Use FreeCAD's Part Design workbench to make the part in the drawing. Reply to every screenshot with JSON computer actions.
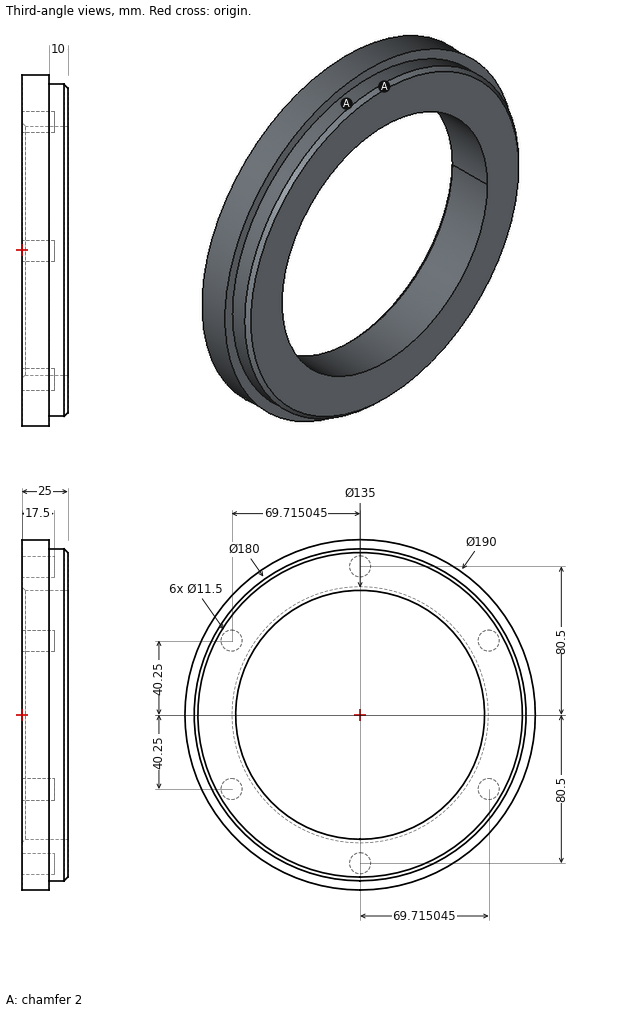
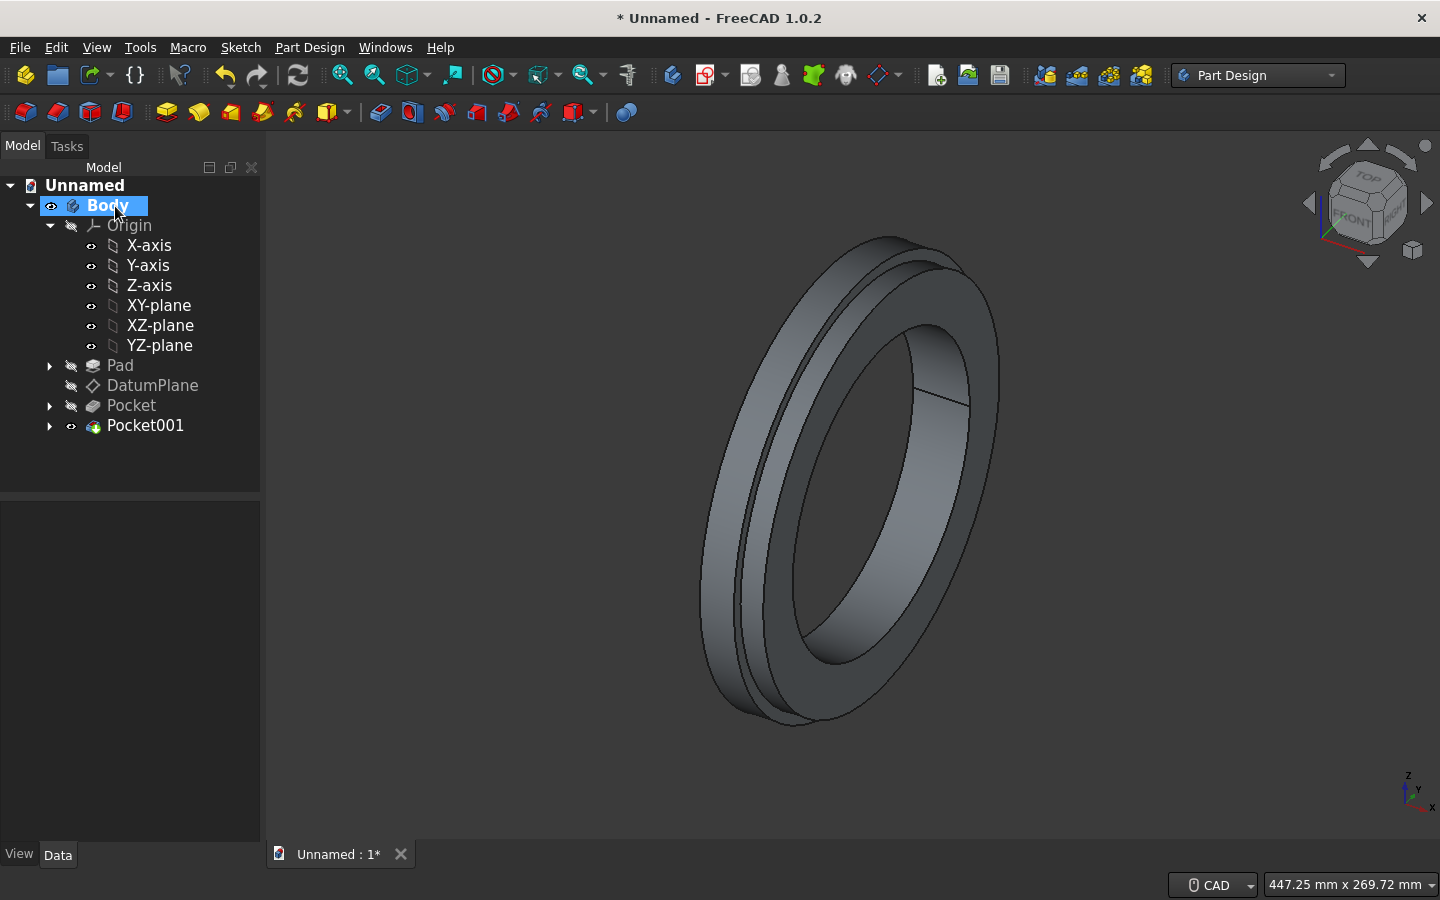
{"action": "left_click", "coordinate": [763, 611]}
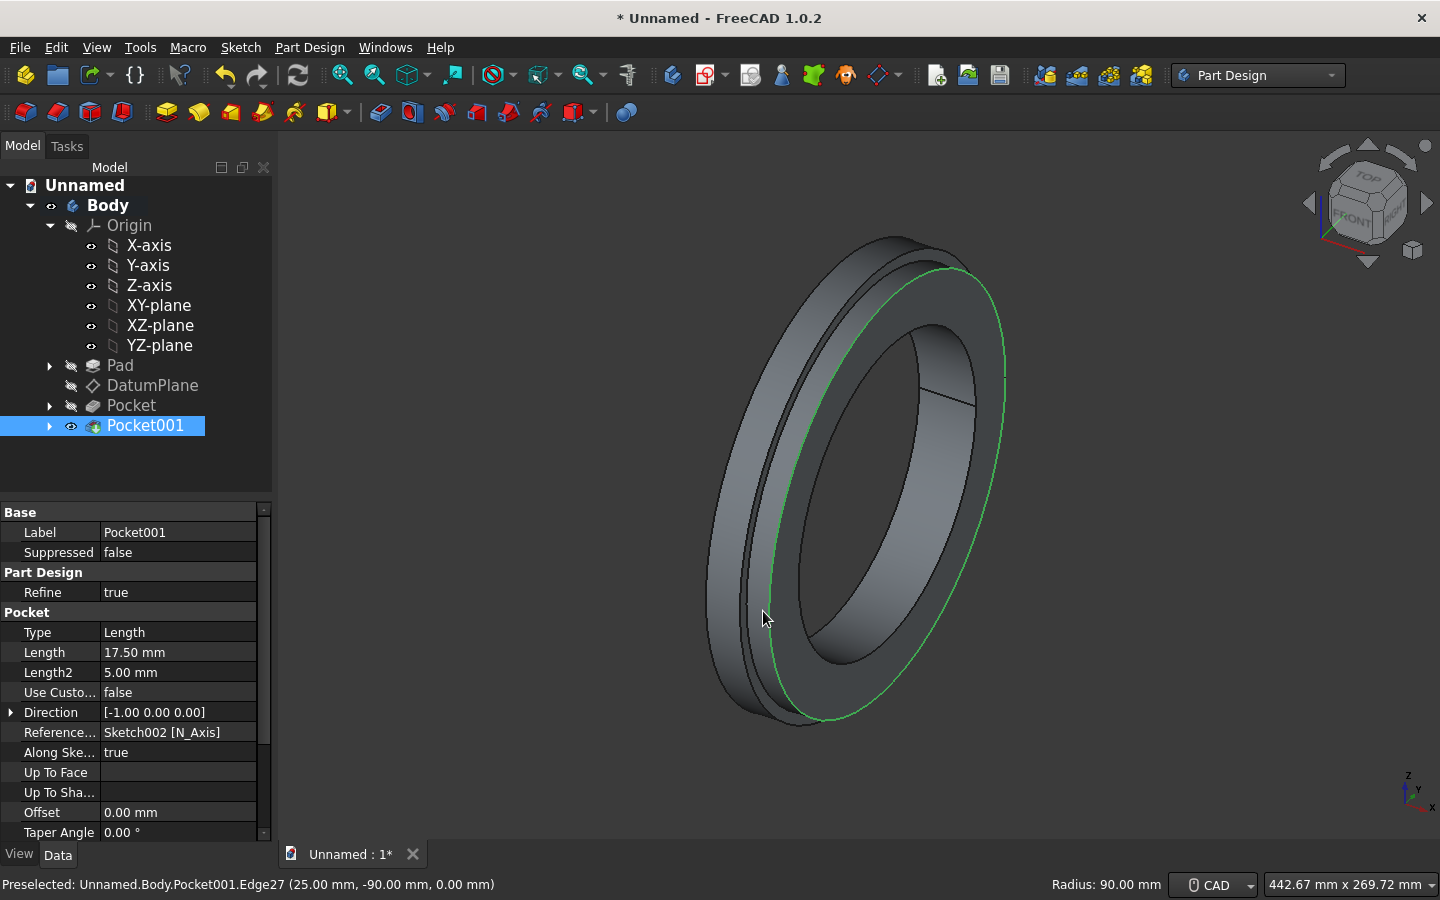
{"action": "key", "text": "0"}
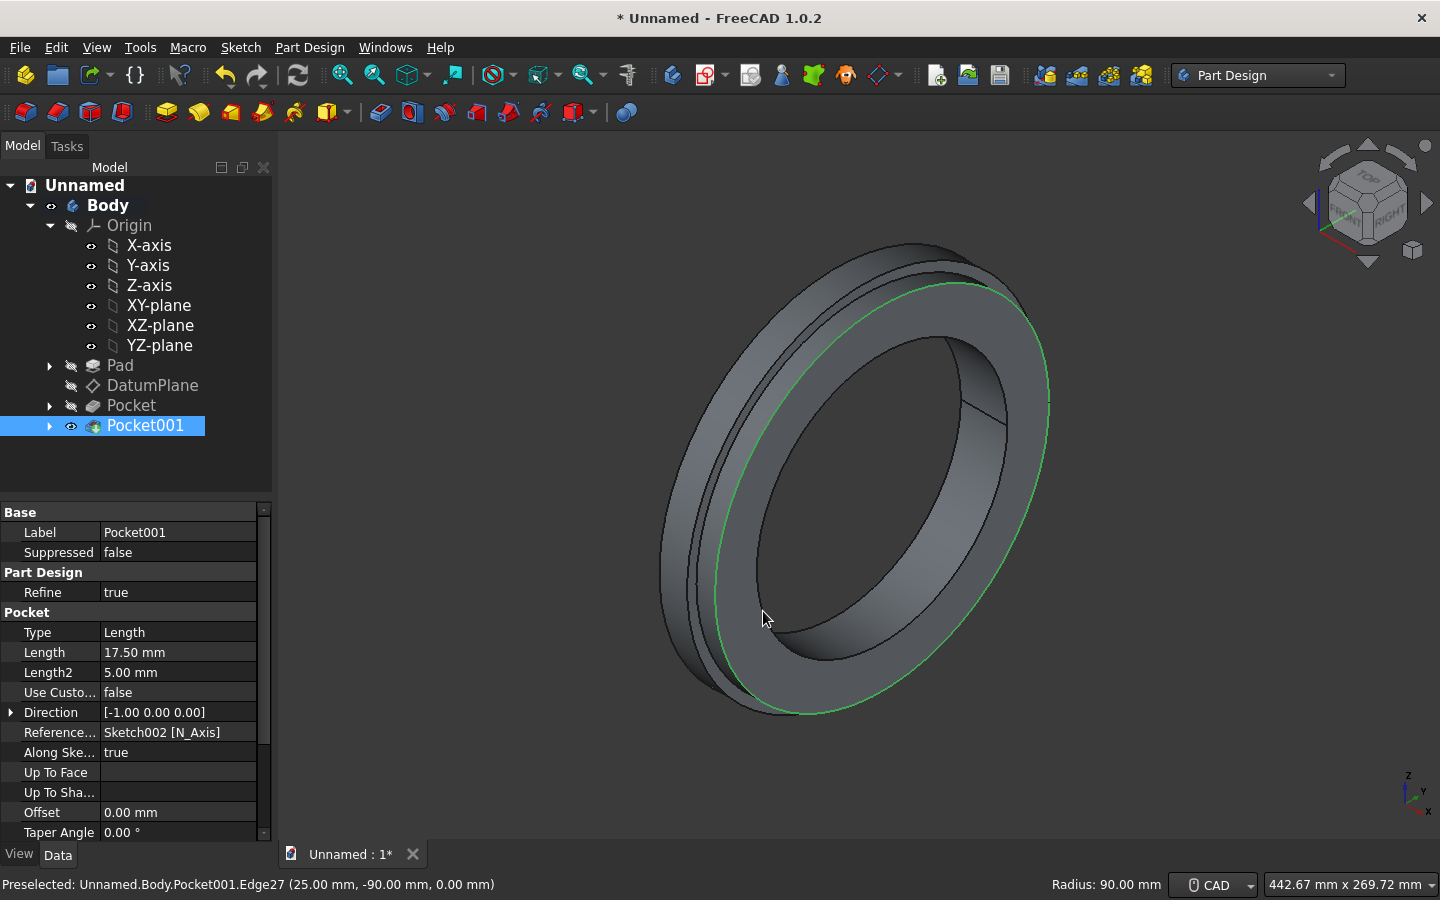
{"action": "key", "text": "2"}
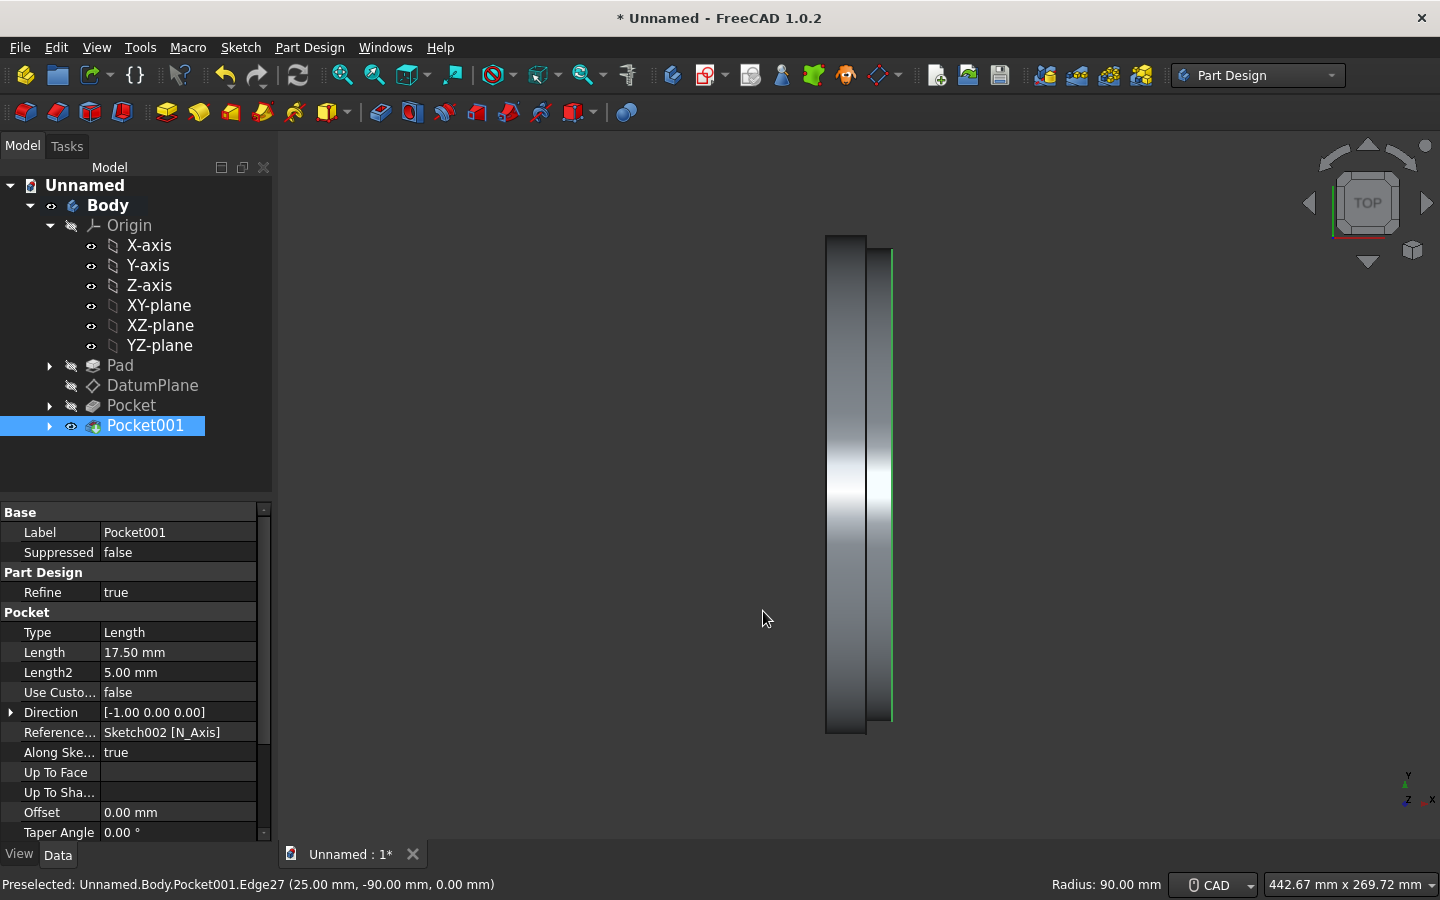
{"action": "key", "text": "1"}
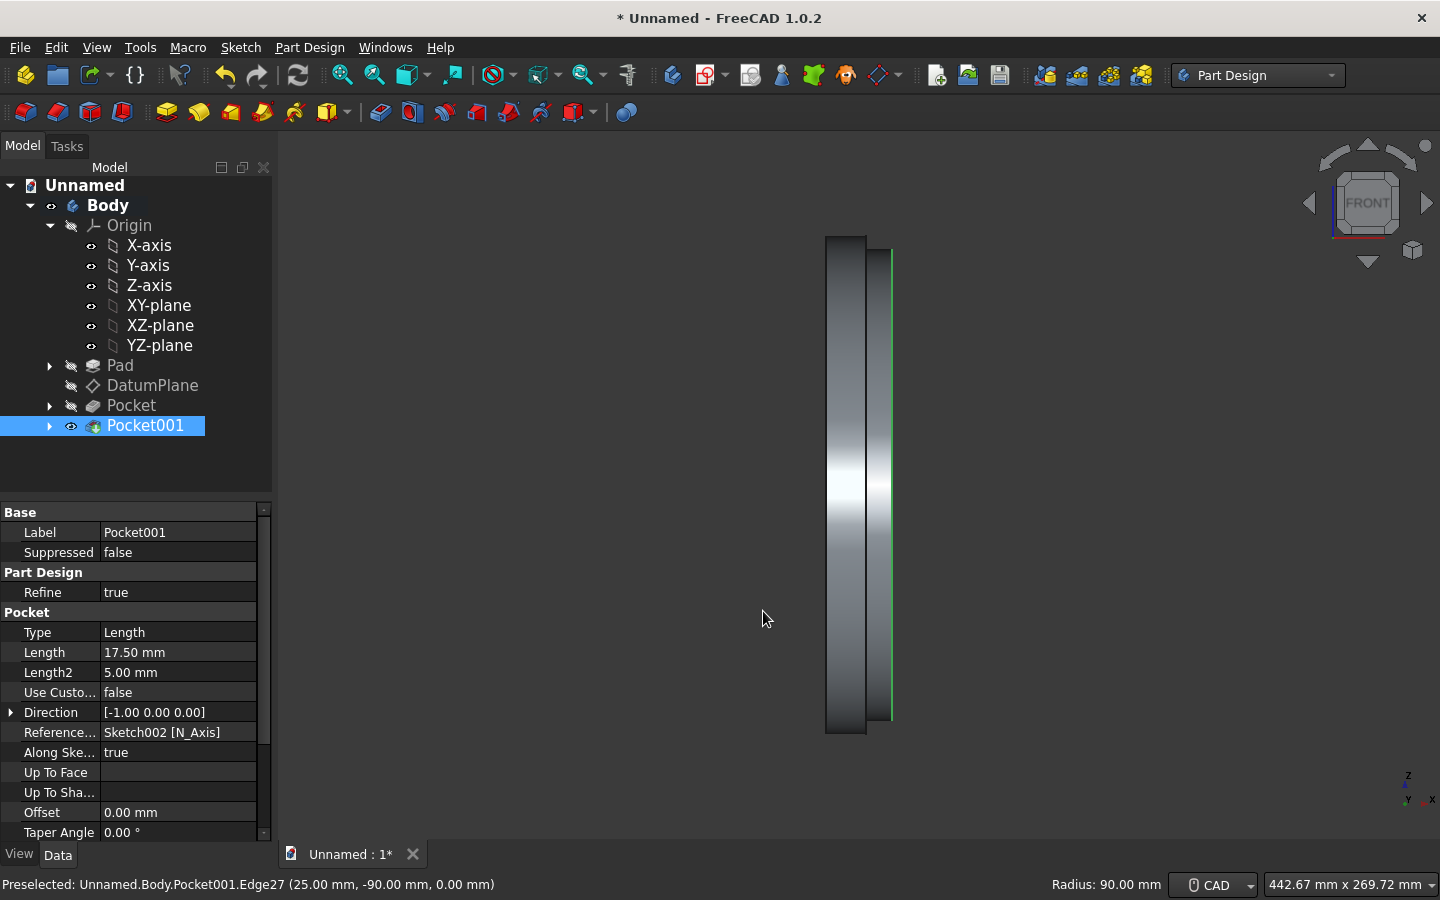
{"action": "key", "text": "3"}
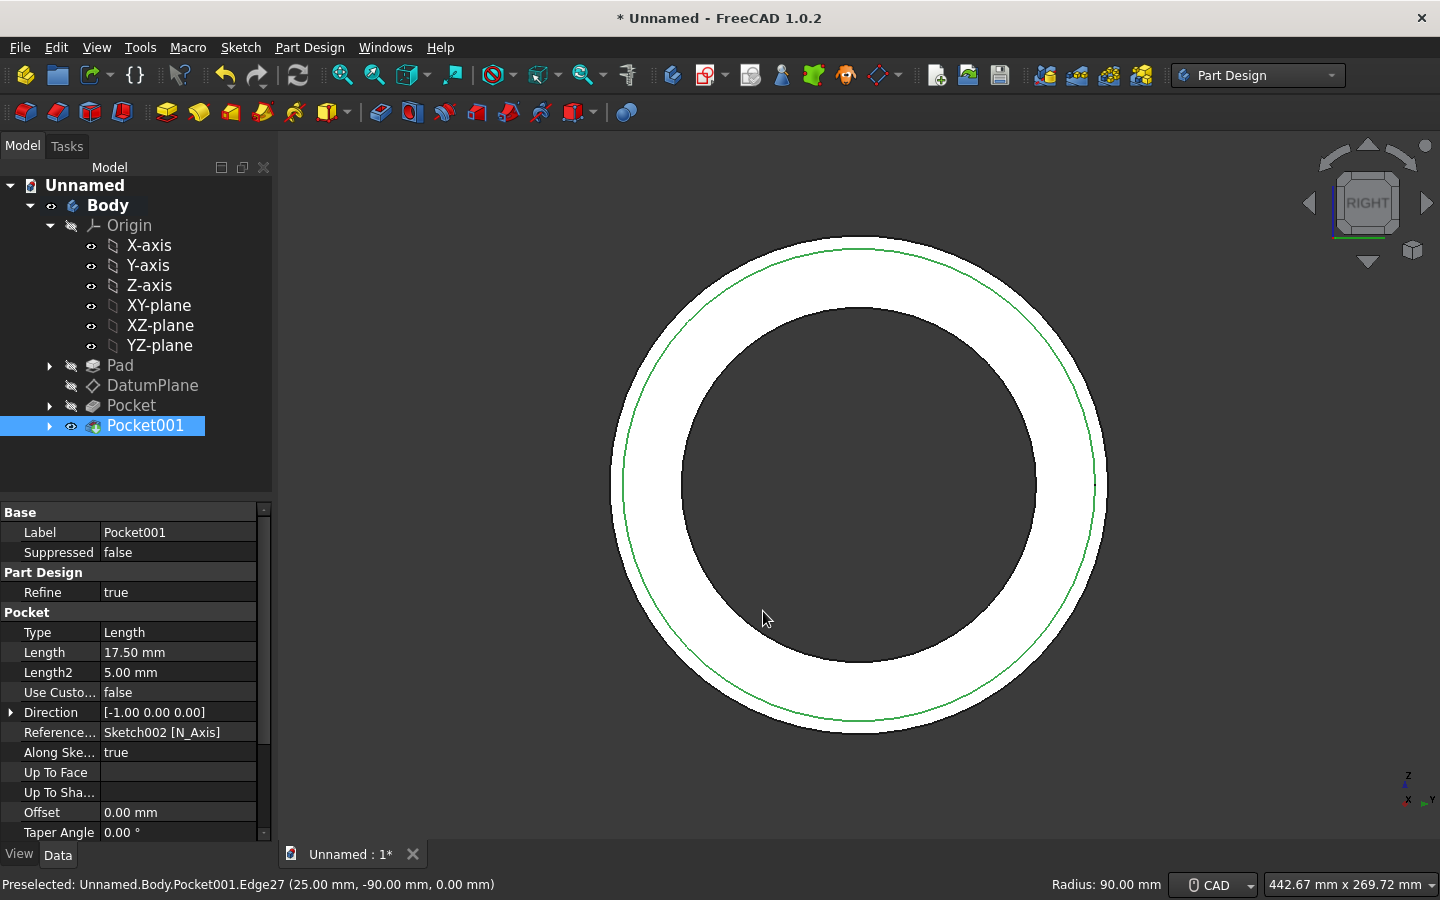
{"action": "key", "text": "5"}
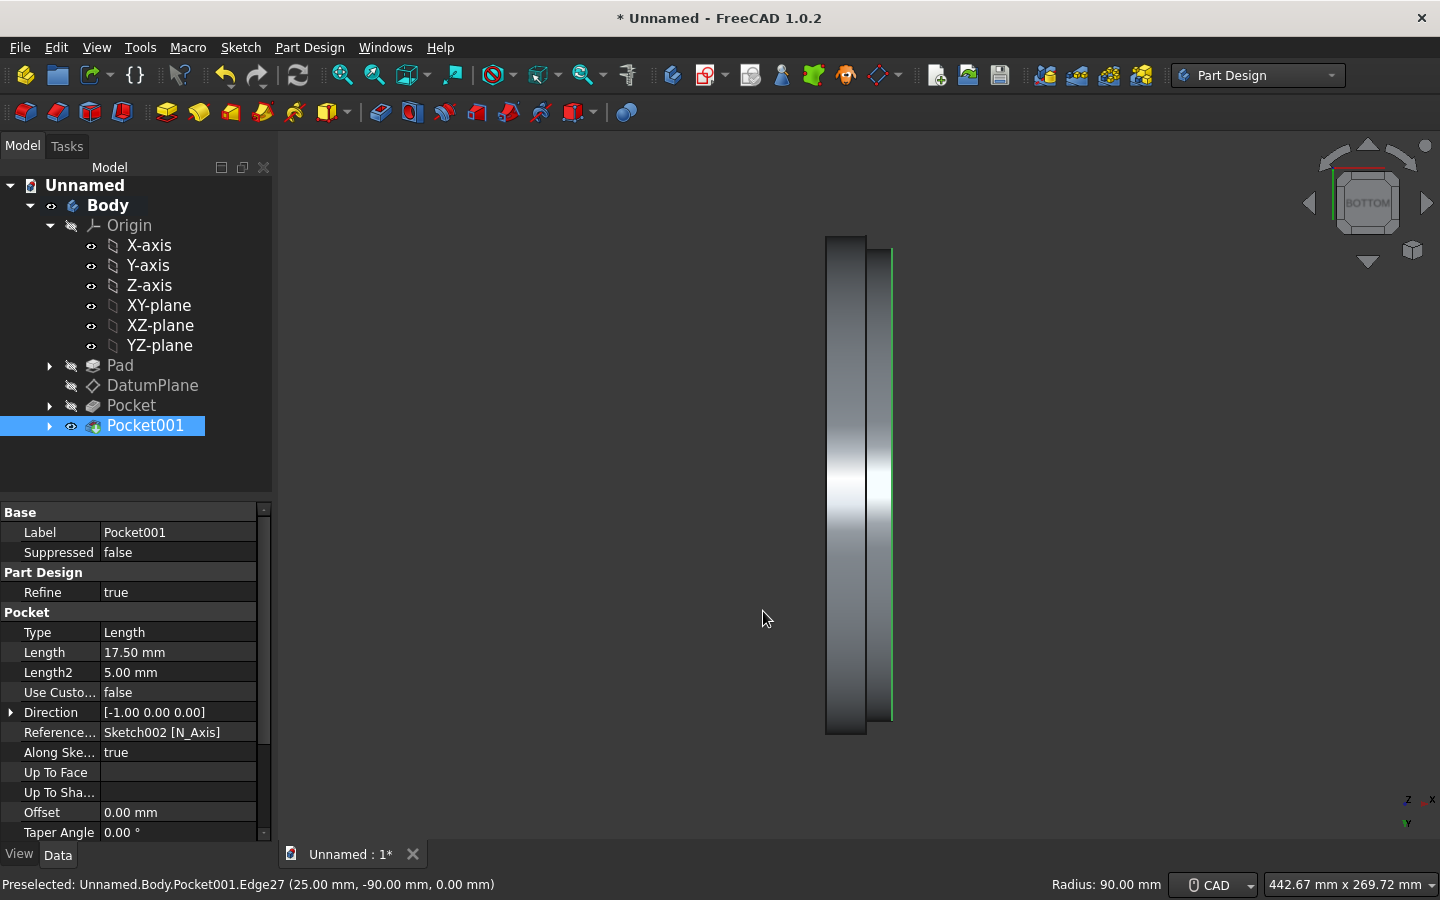
{"action": "key", "text": "4"}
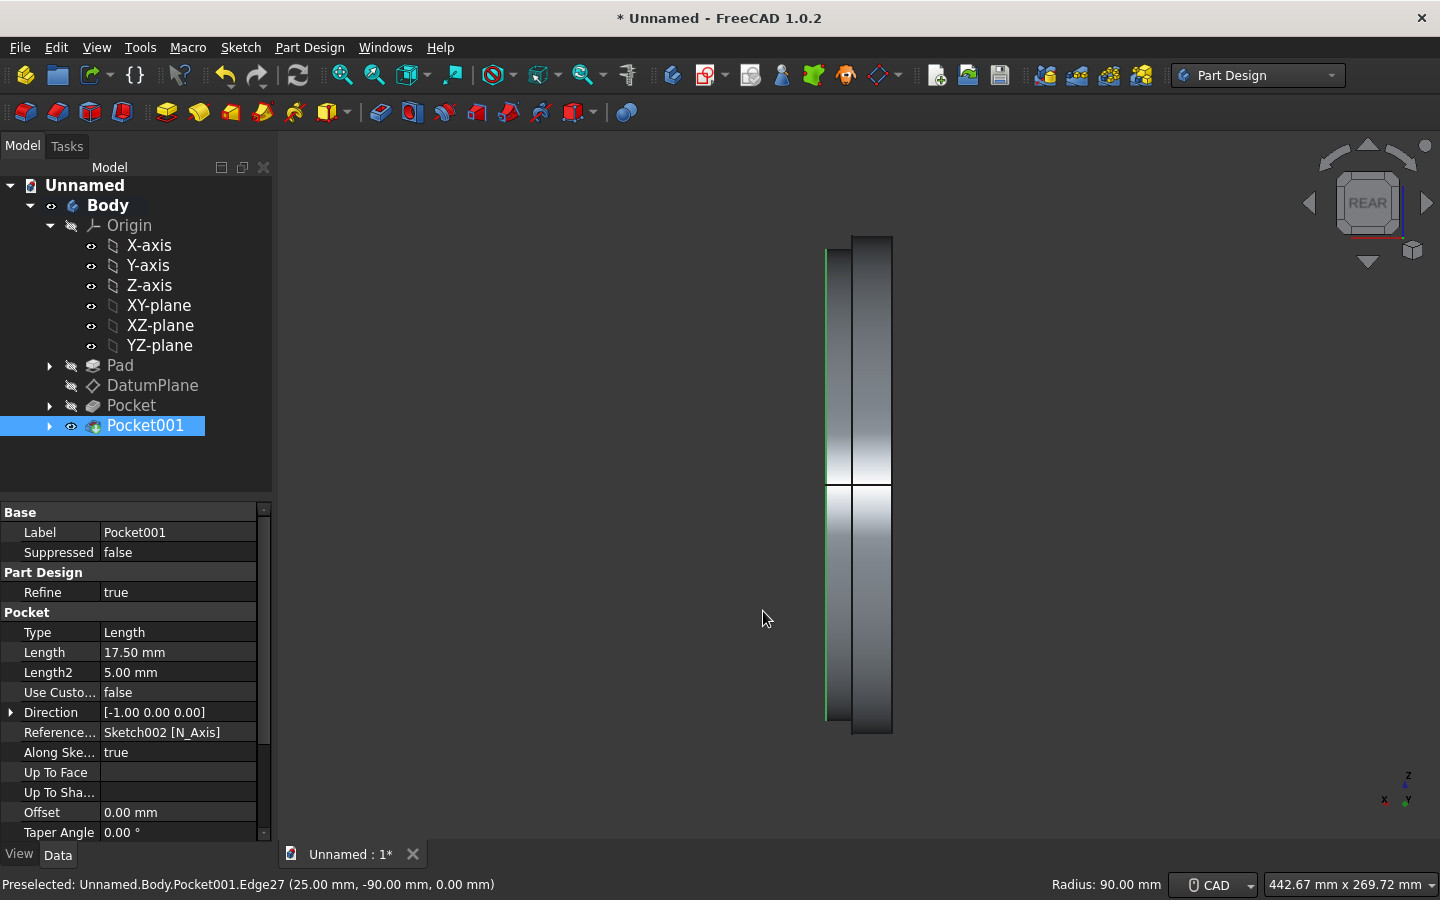
{"action": "key", "text": "6"}